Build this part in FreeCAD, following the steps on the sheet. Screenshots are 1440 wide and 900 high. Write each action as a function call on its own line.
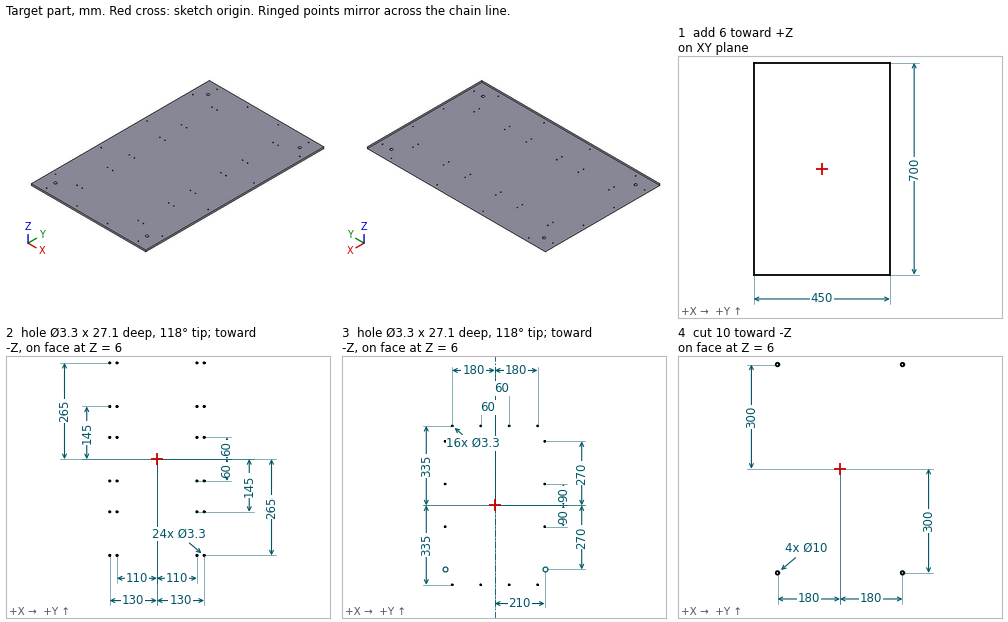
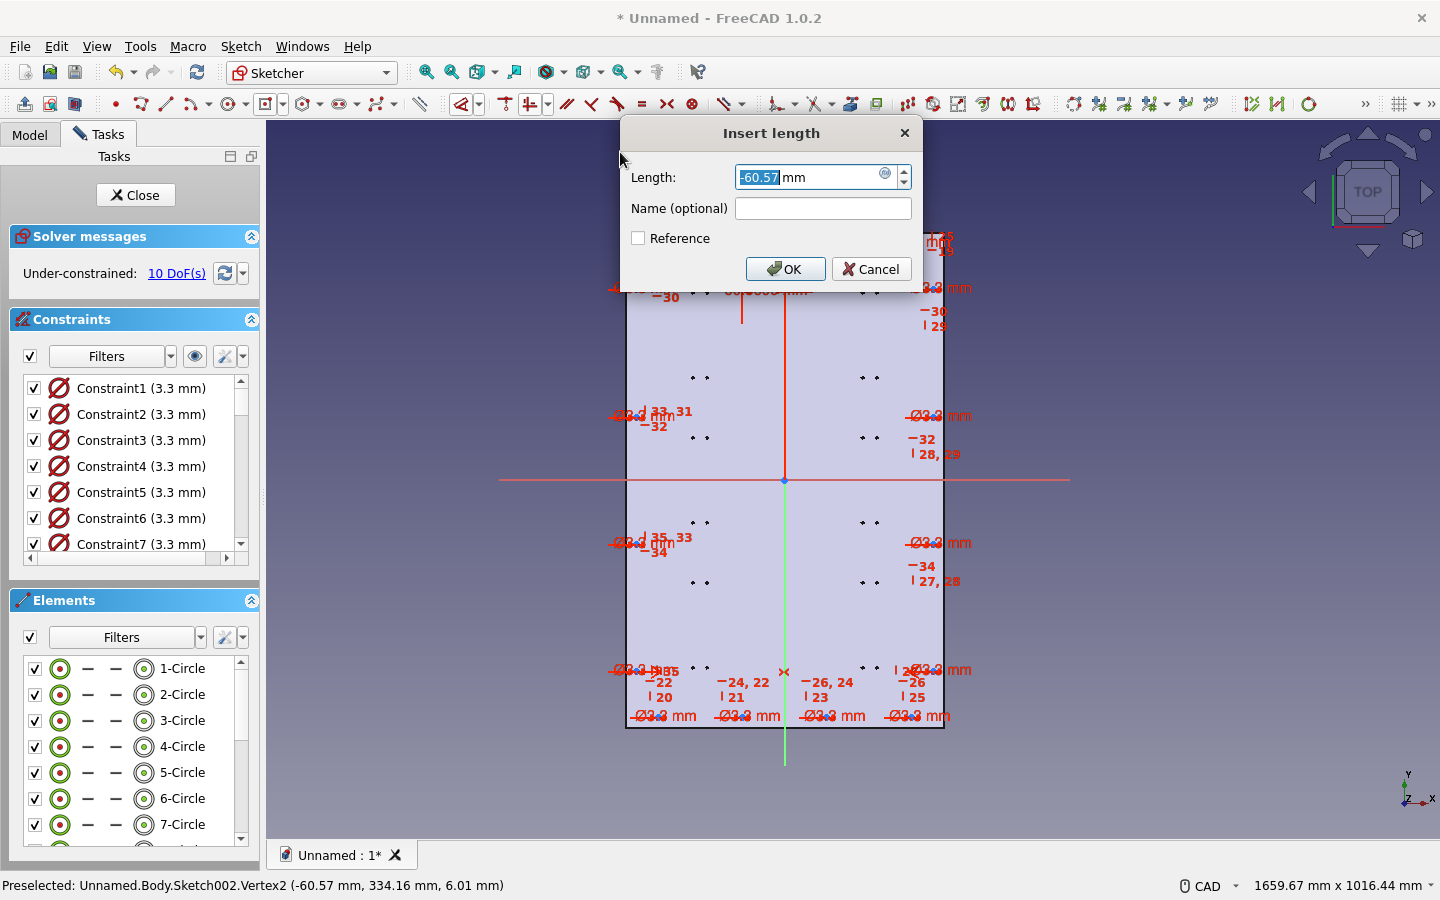
text(-60)
key(Return)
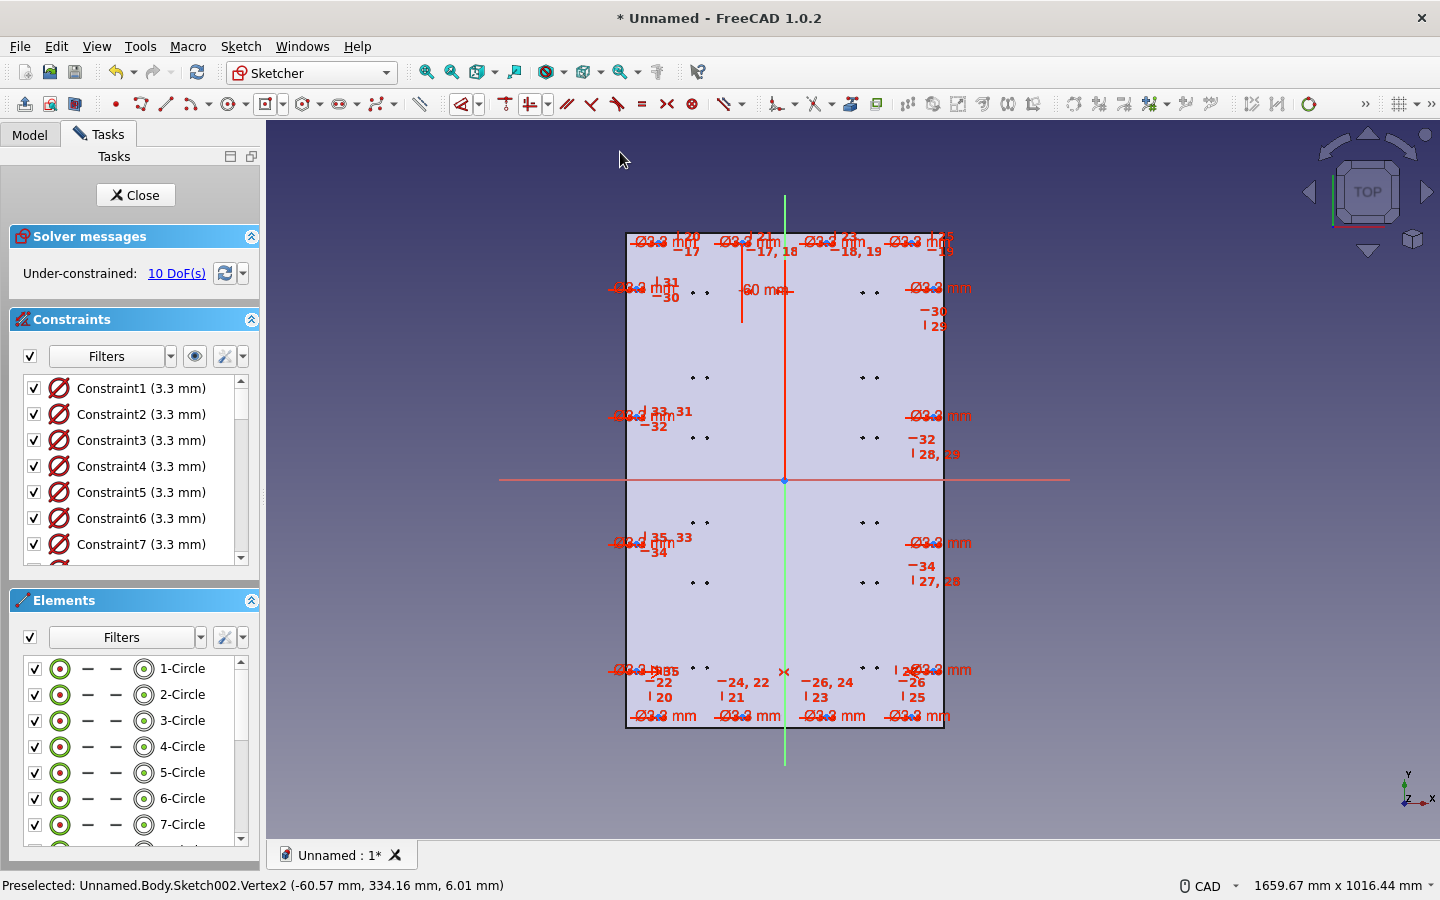
click(827, 244)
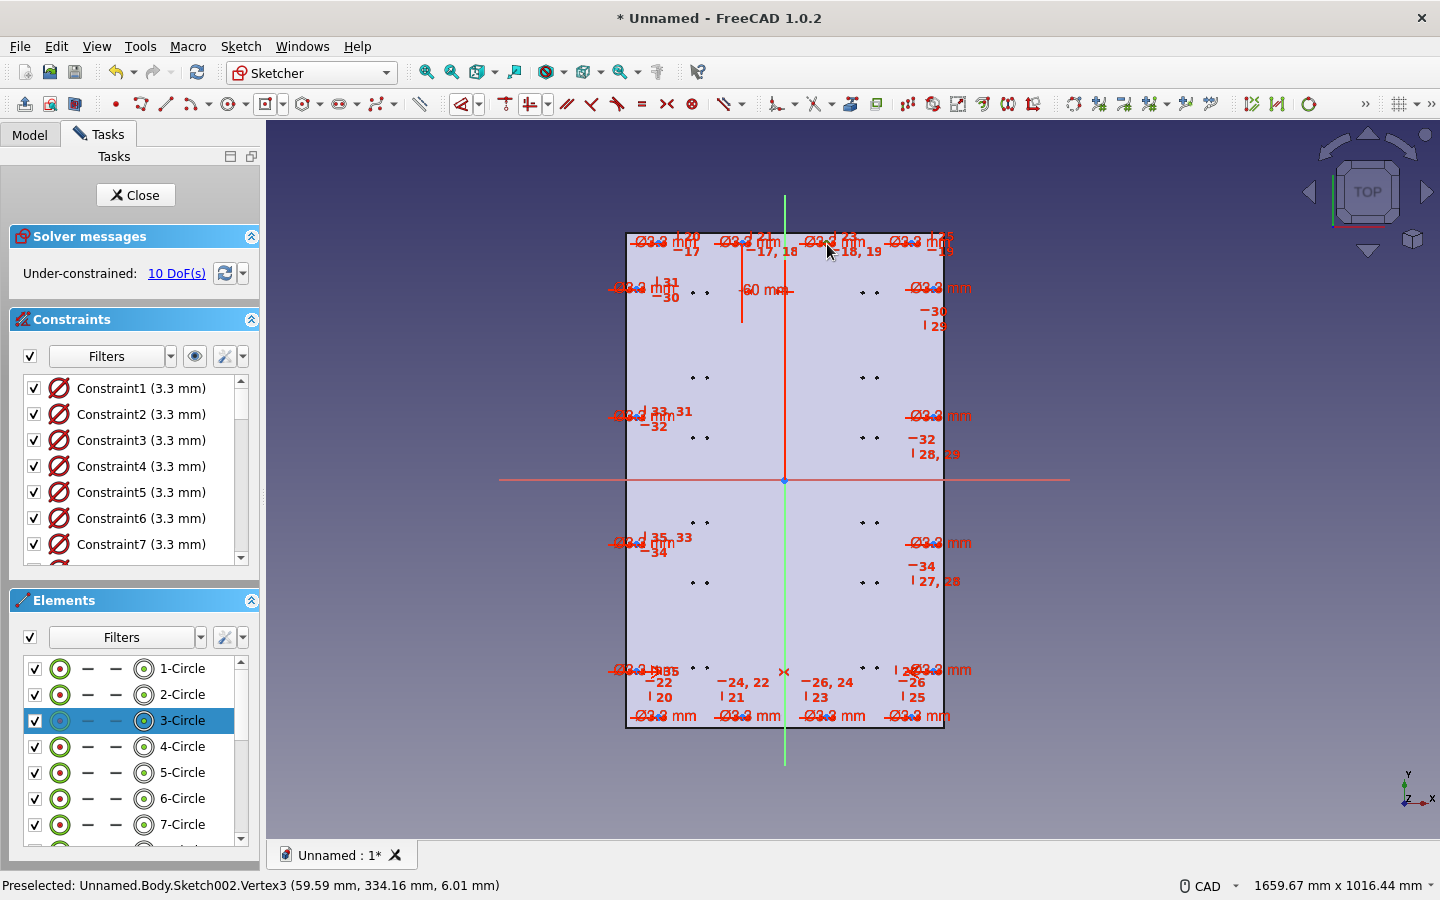
click(478, 104)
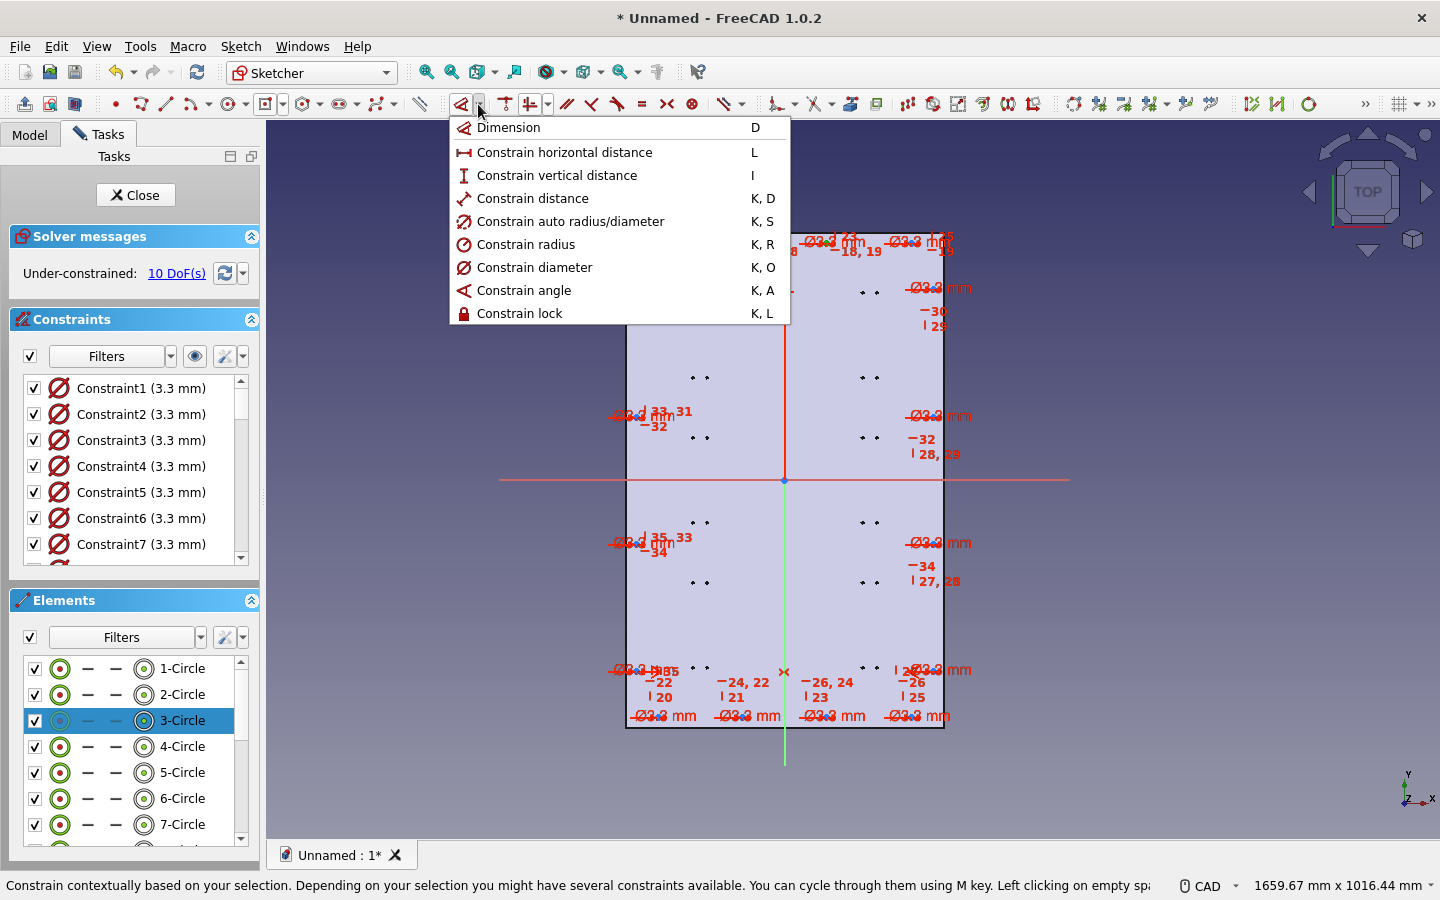
click(620, 152)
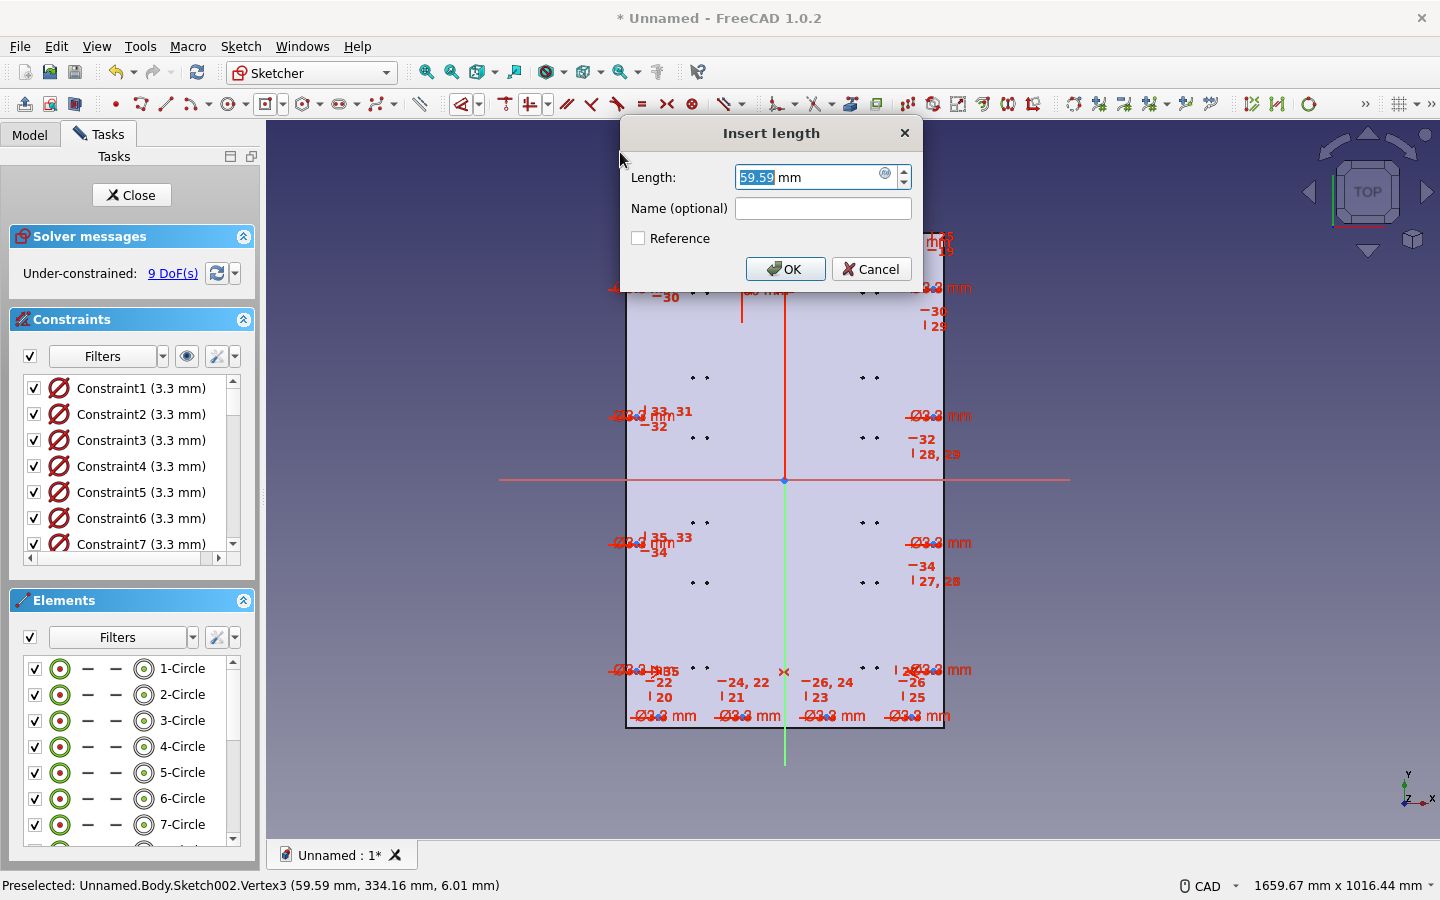
text(60)
key(Return)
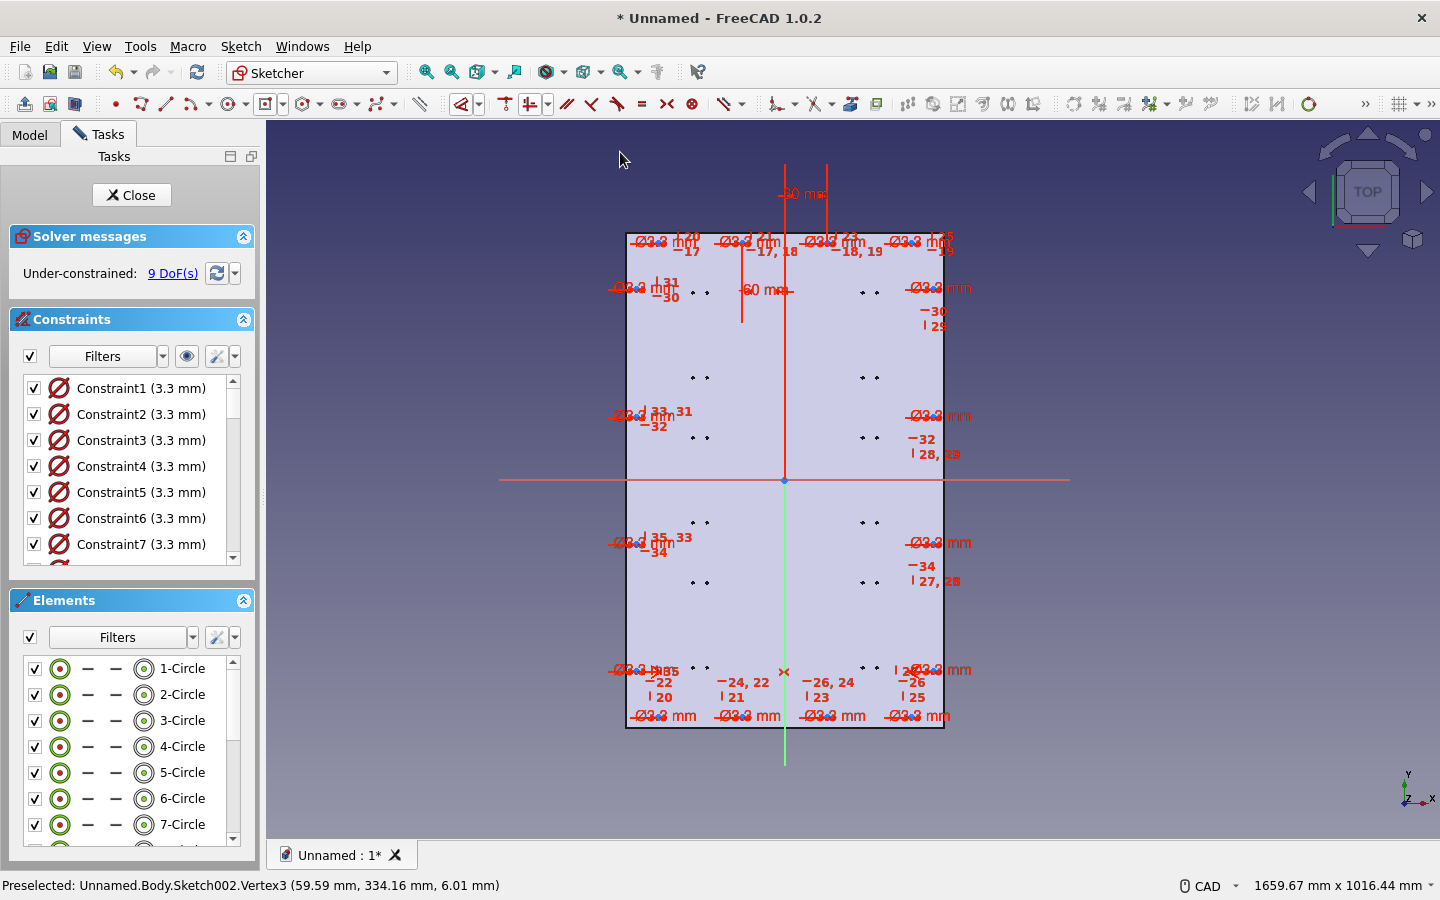
click(933, 545)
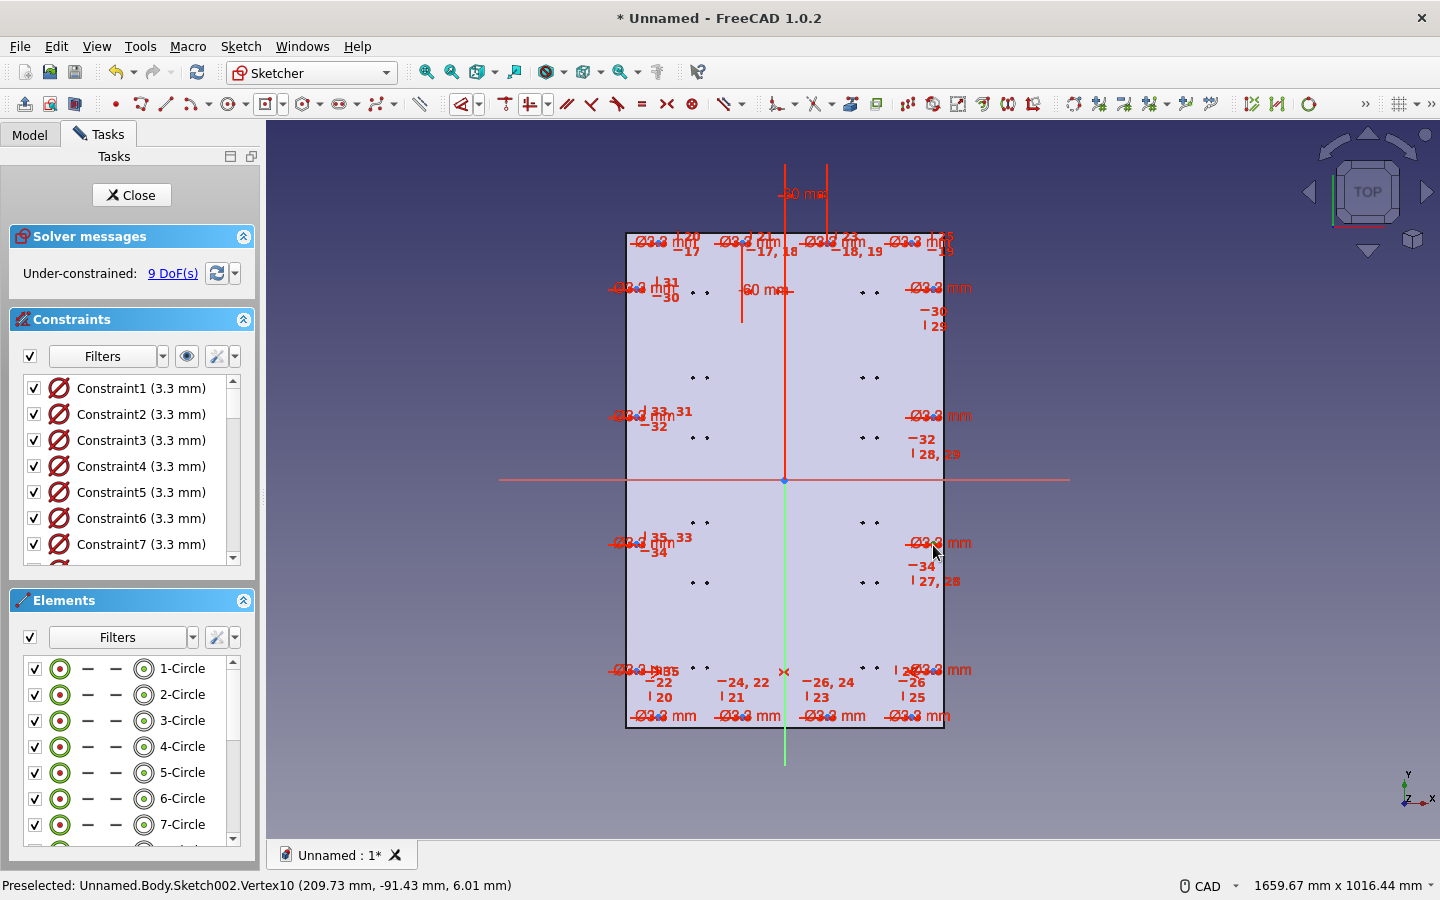
click(478, 104)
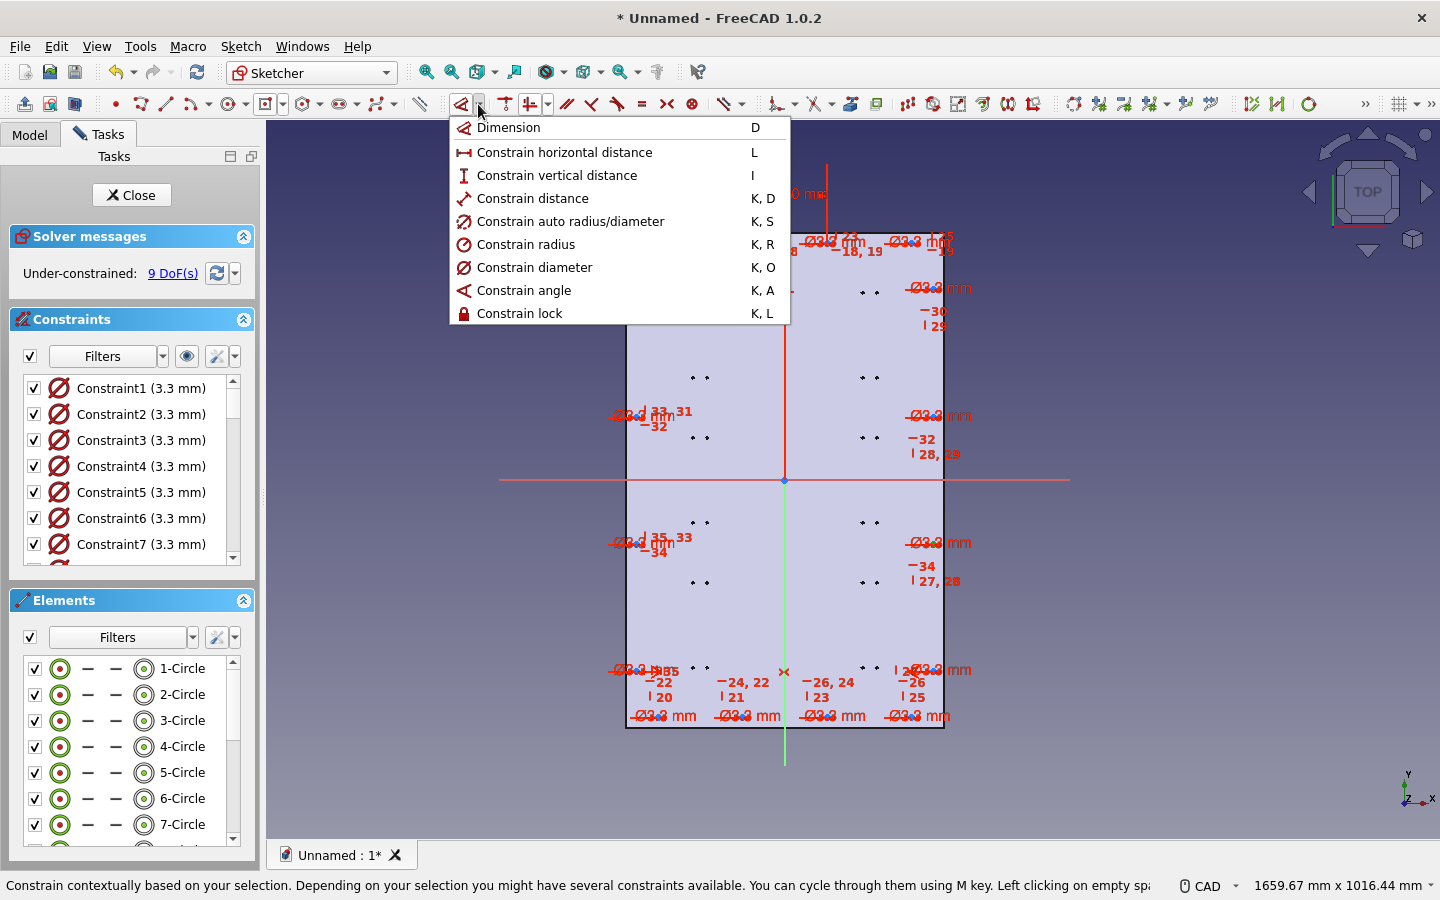
click(620, 176)